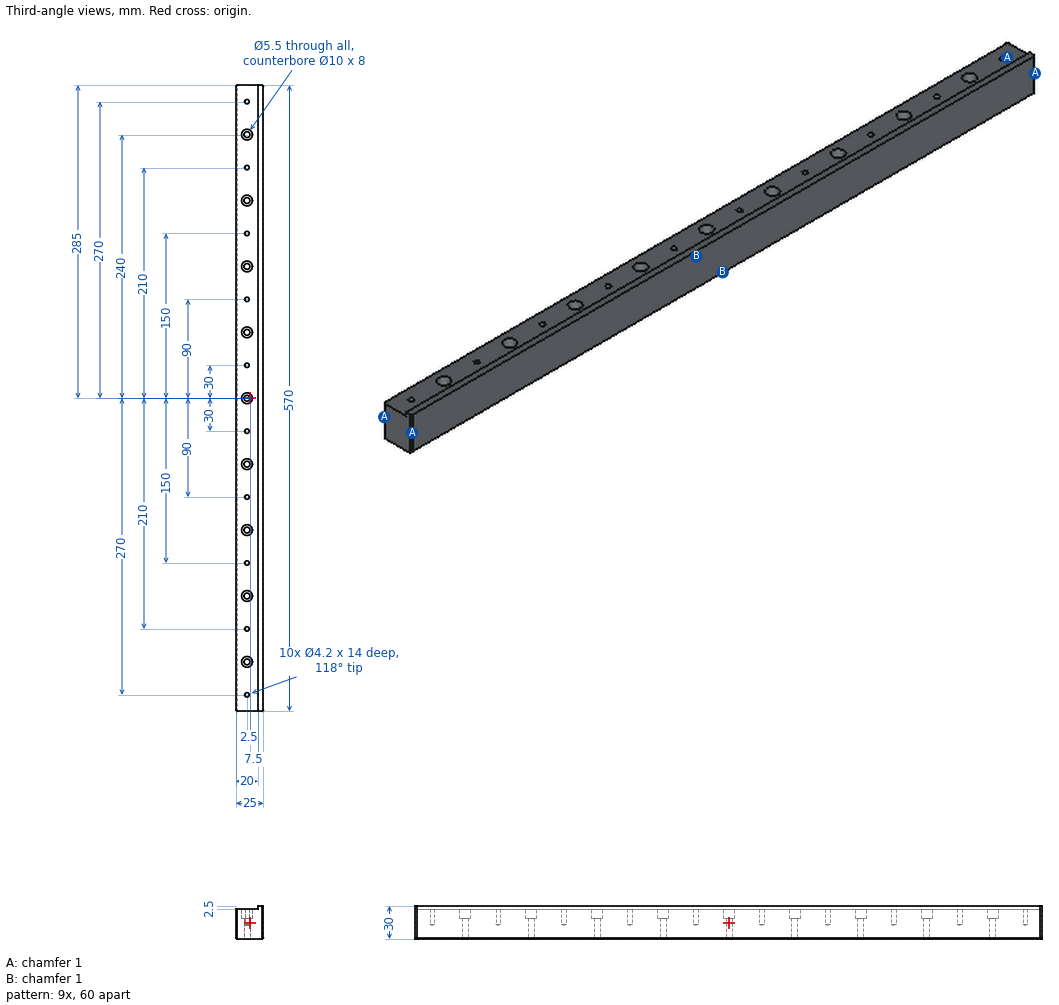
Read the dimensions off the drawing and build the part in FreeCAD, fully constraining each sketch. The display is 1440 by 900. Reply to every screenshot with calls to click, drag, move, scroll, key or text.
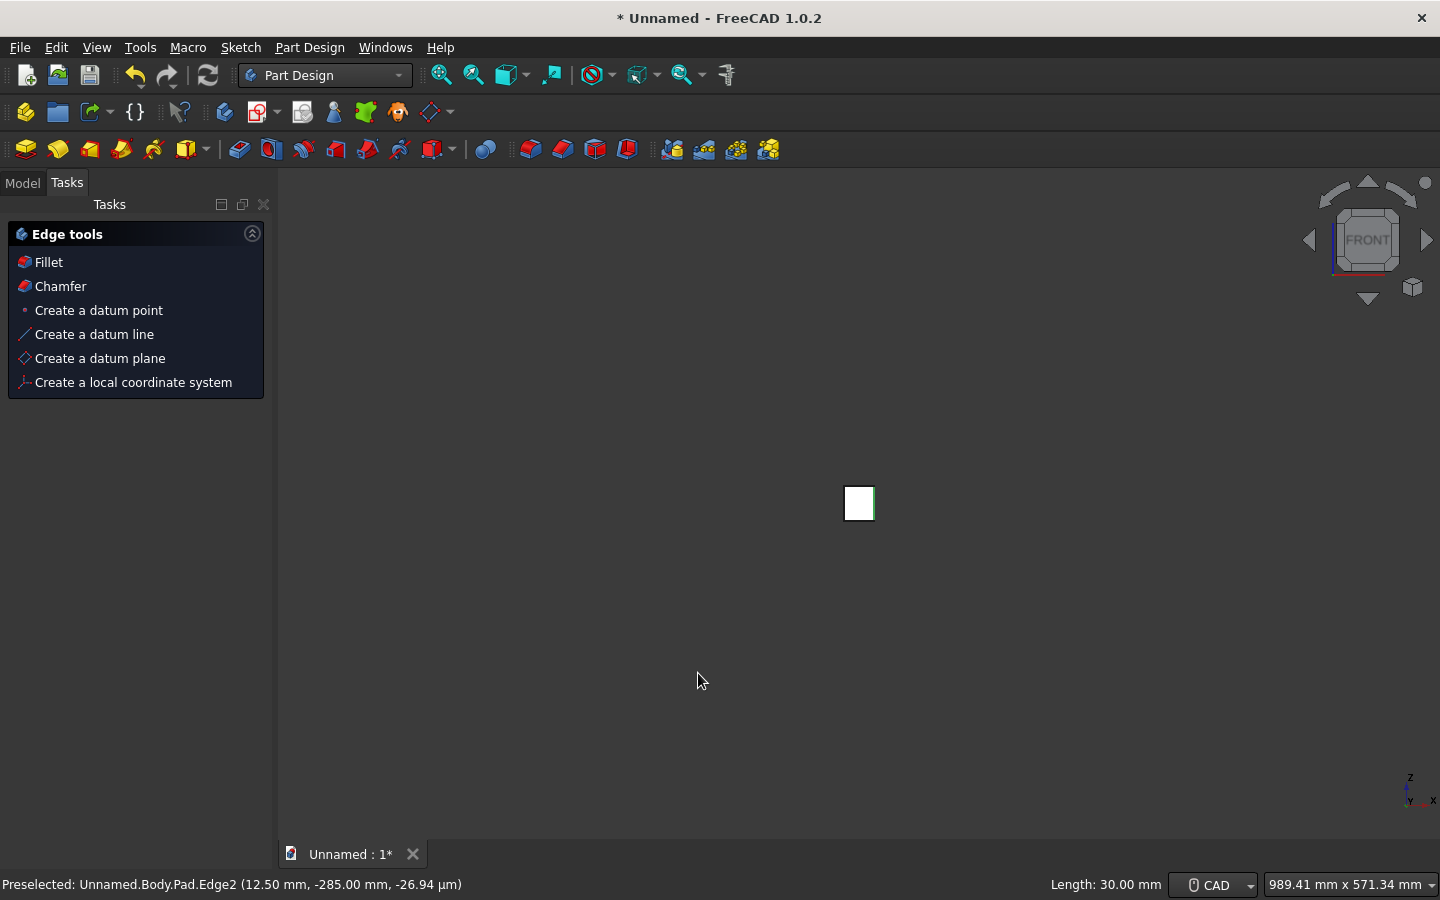
click(442, 76)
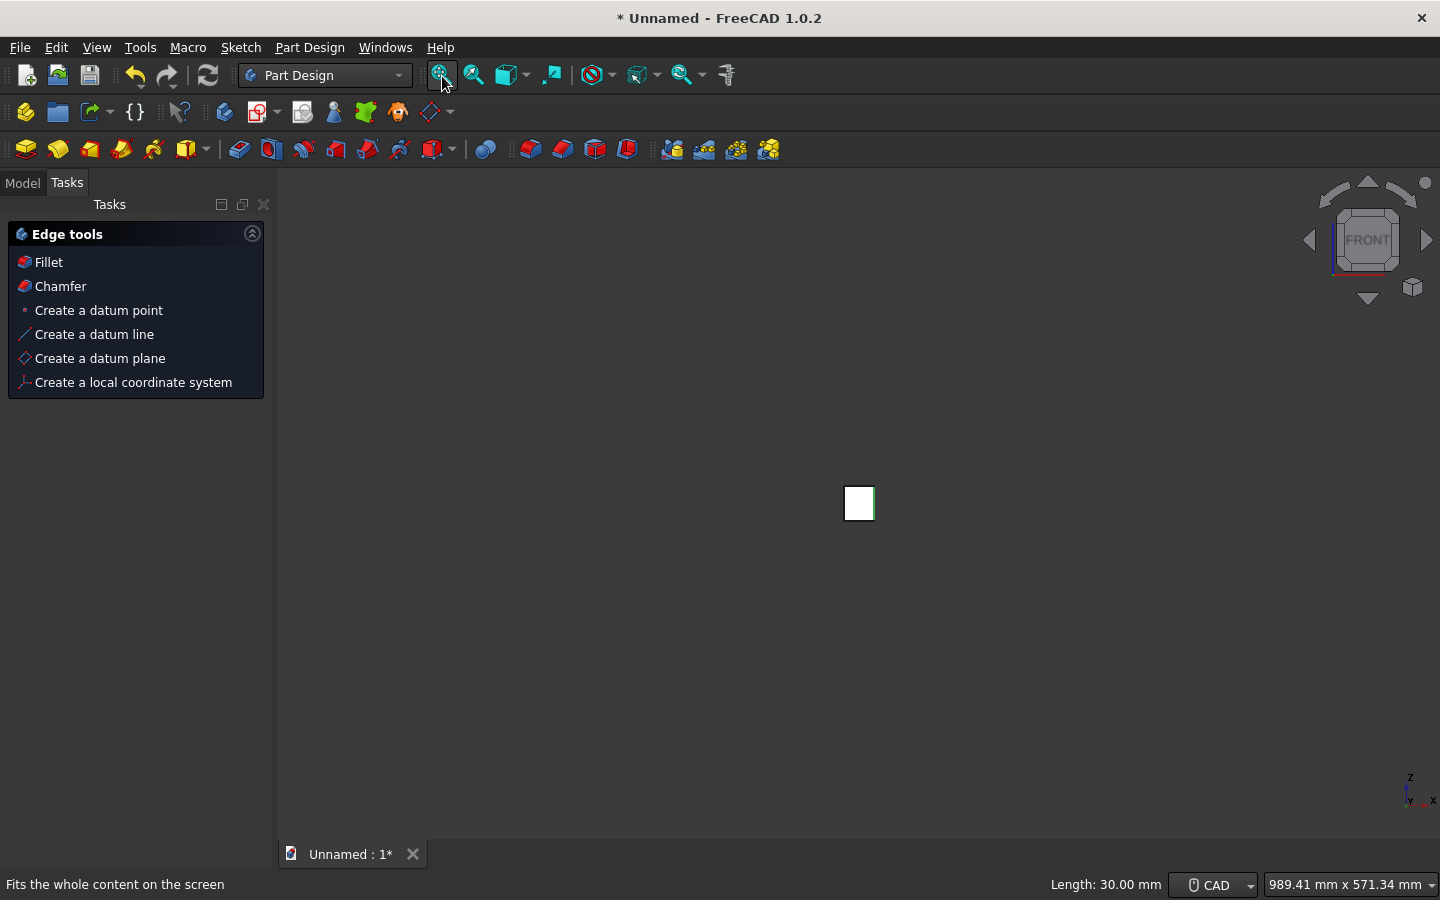
click(844, 503, ctrl)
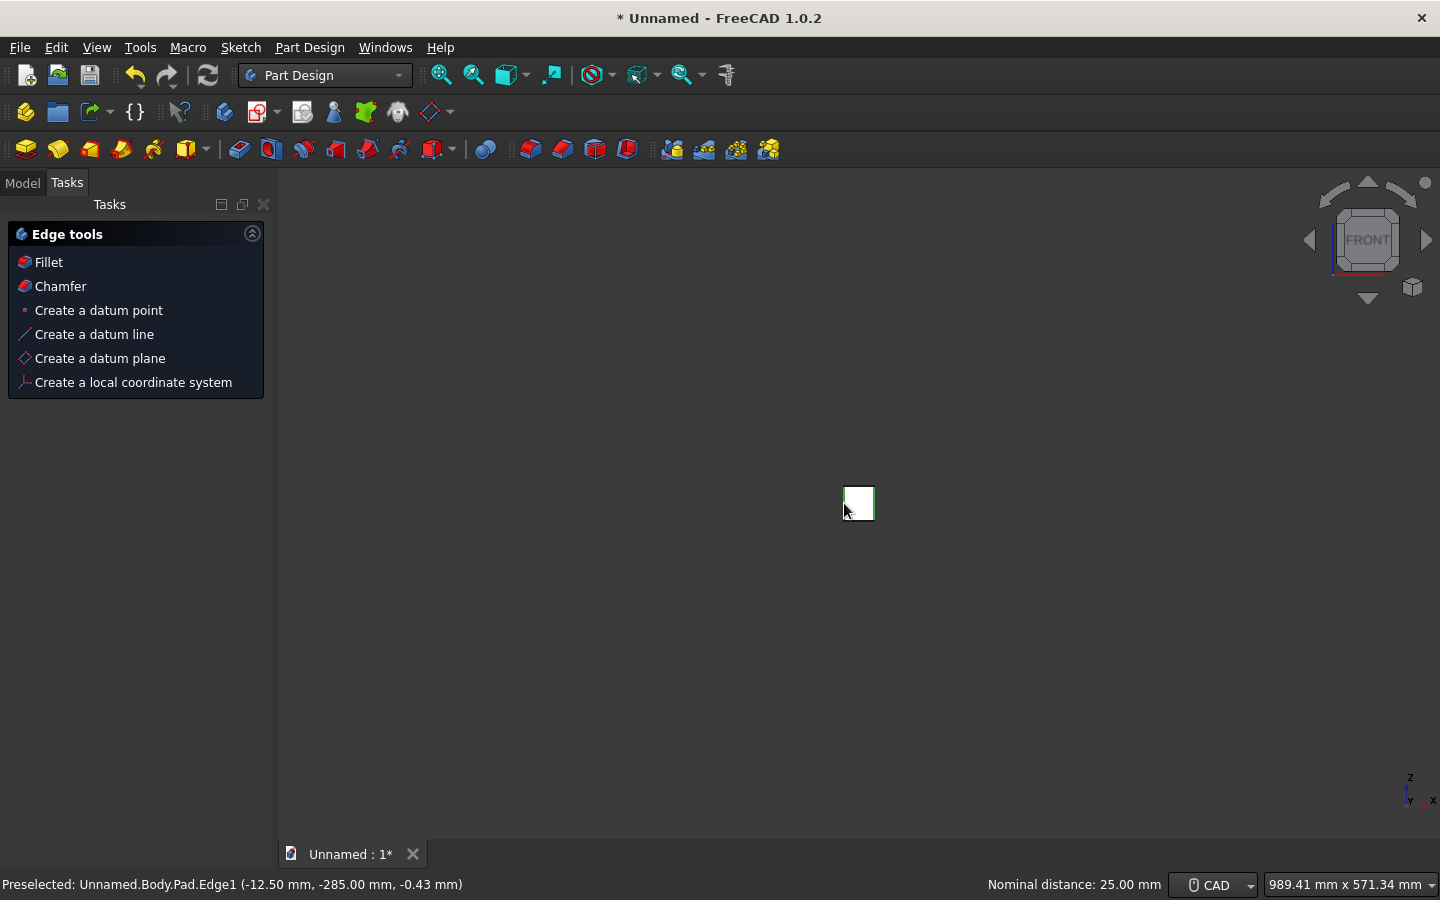
key(3)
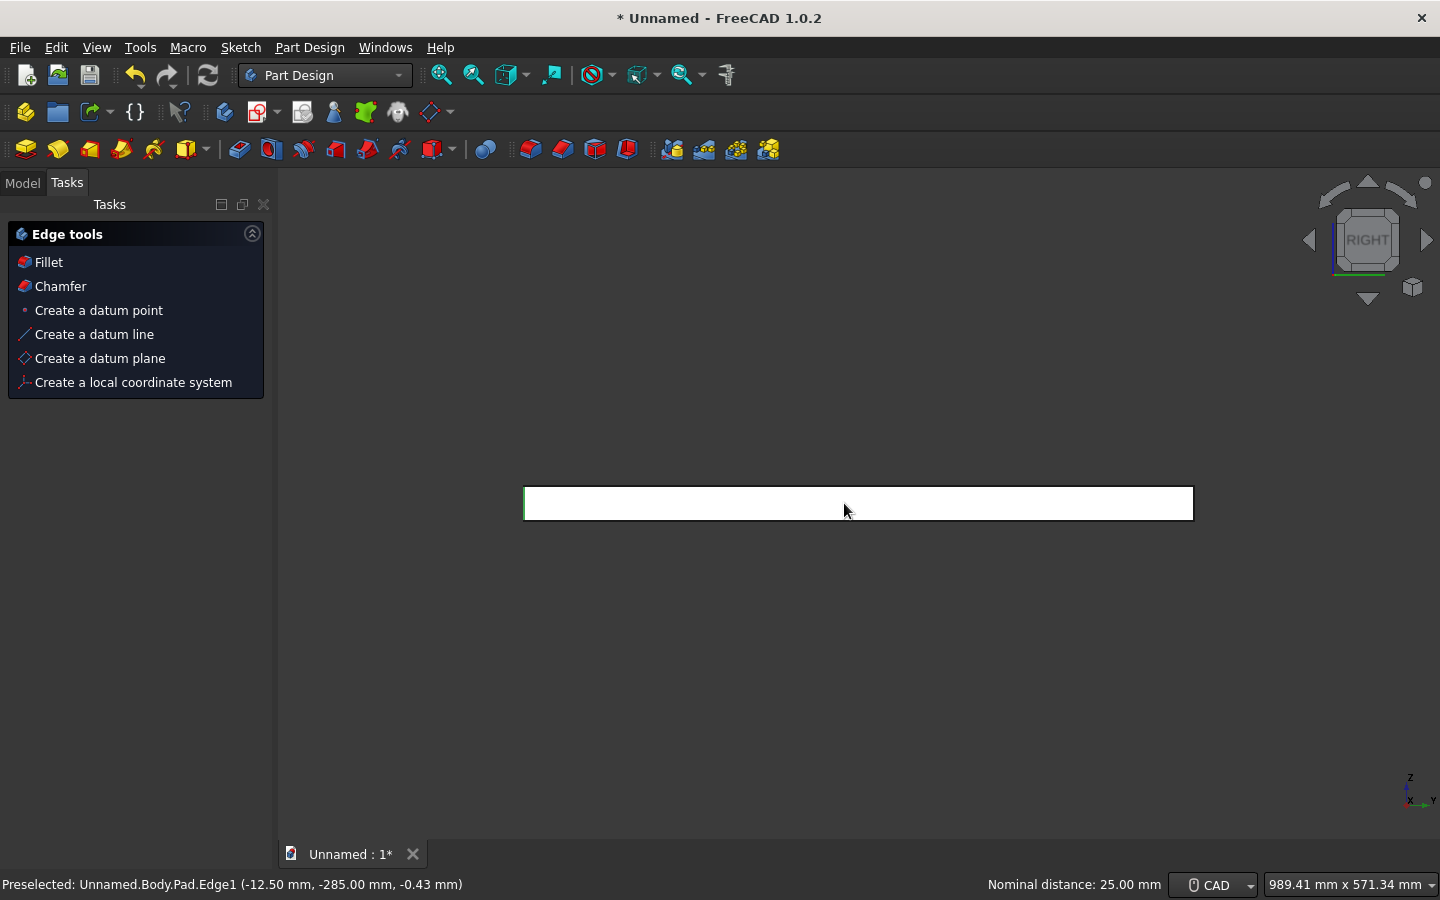
click(1194, 502, ctrl)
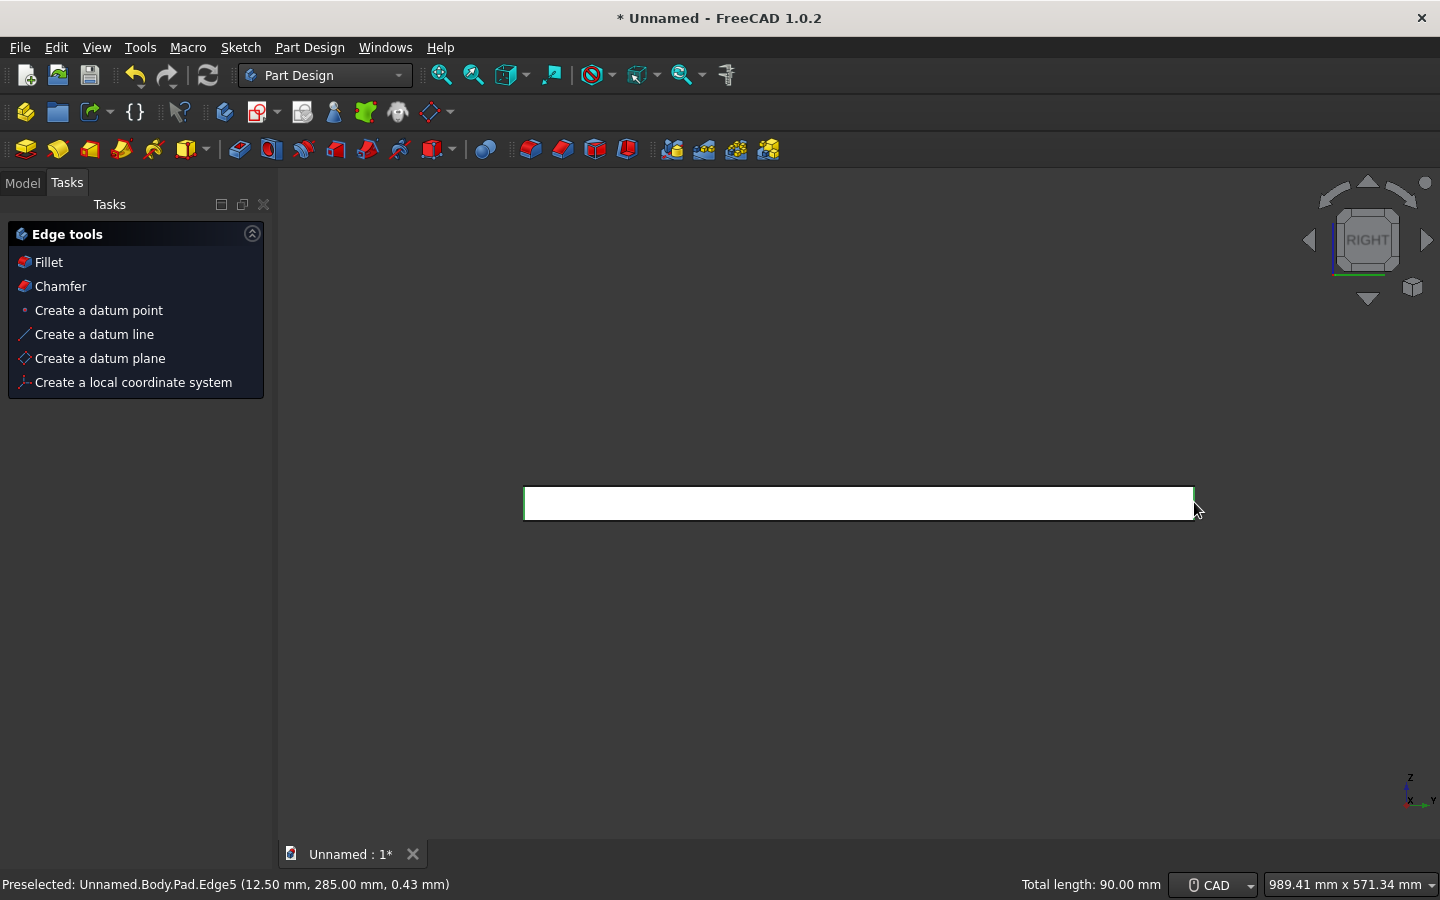
key(5)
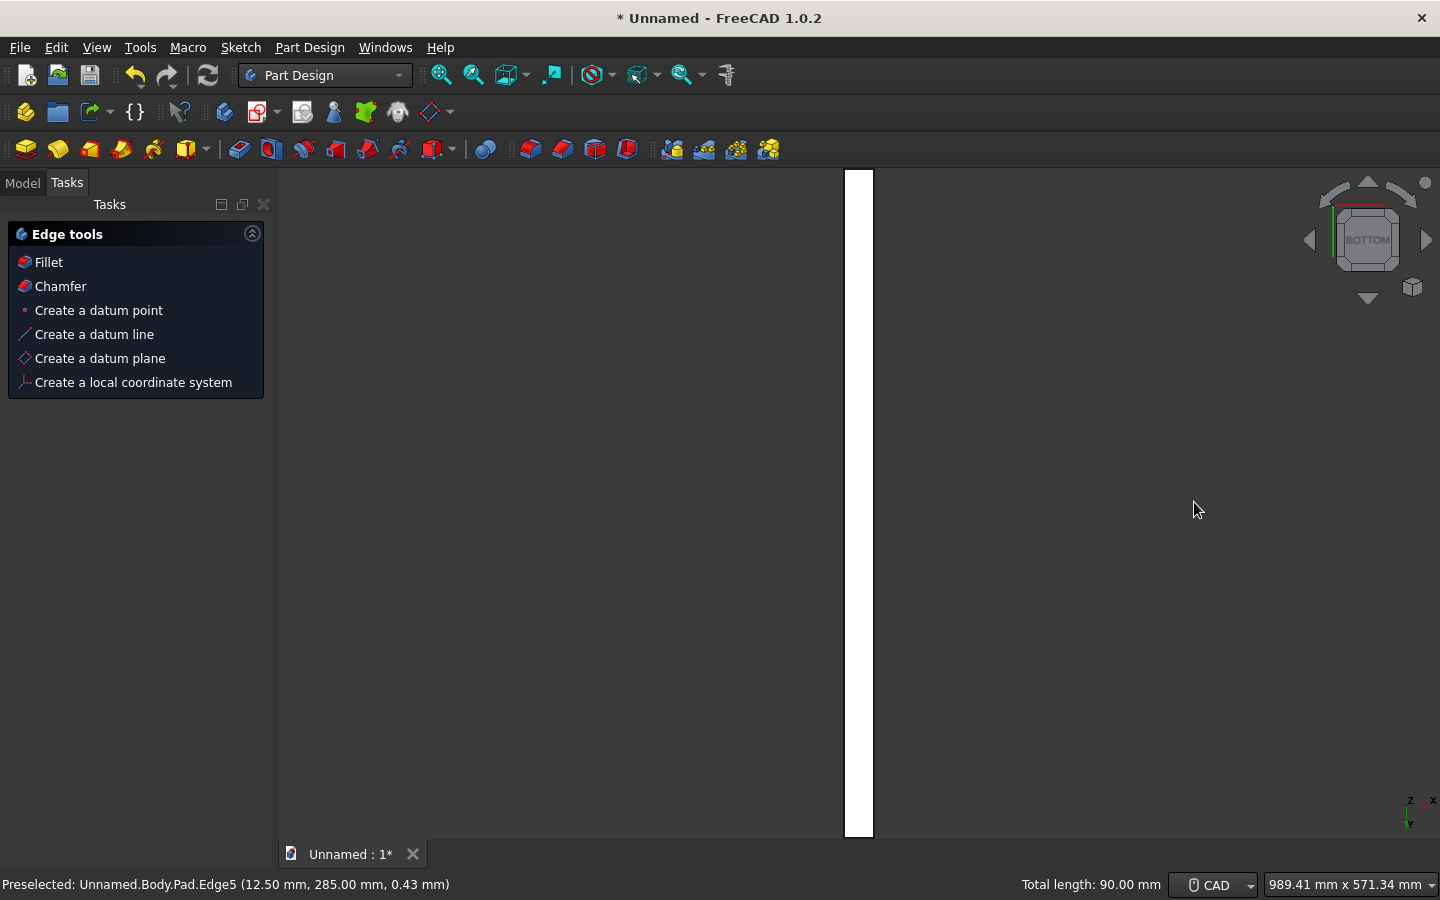
key(4)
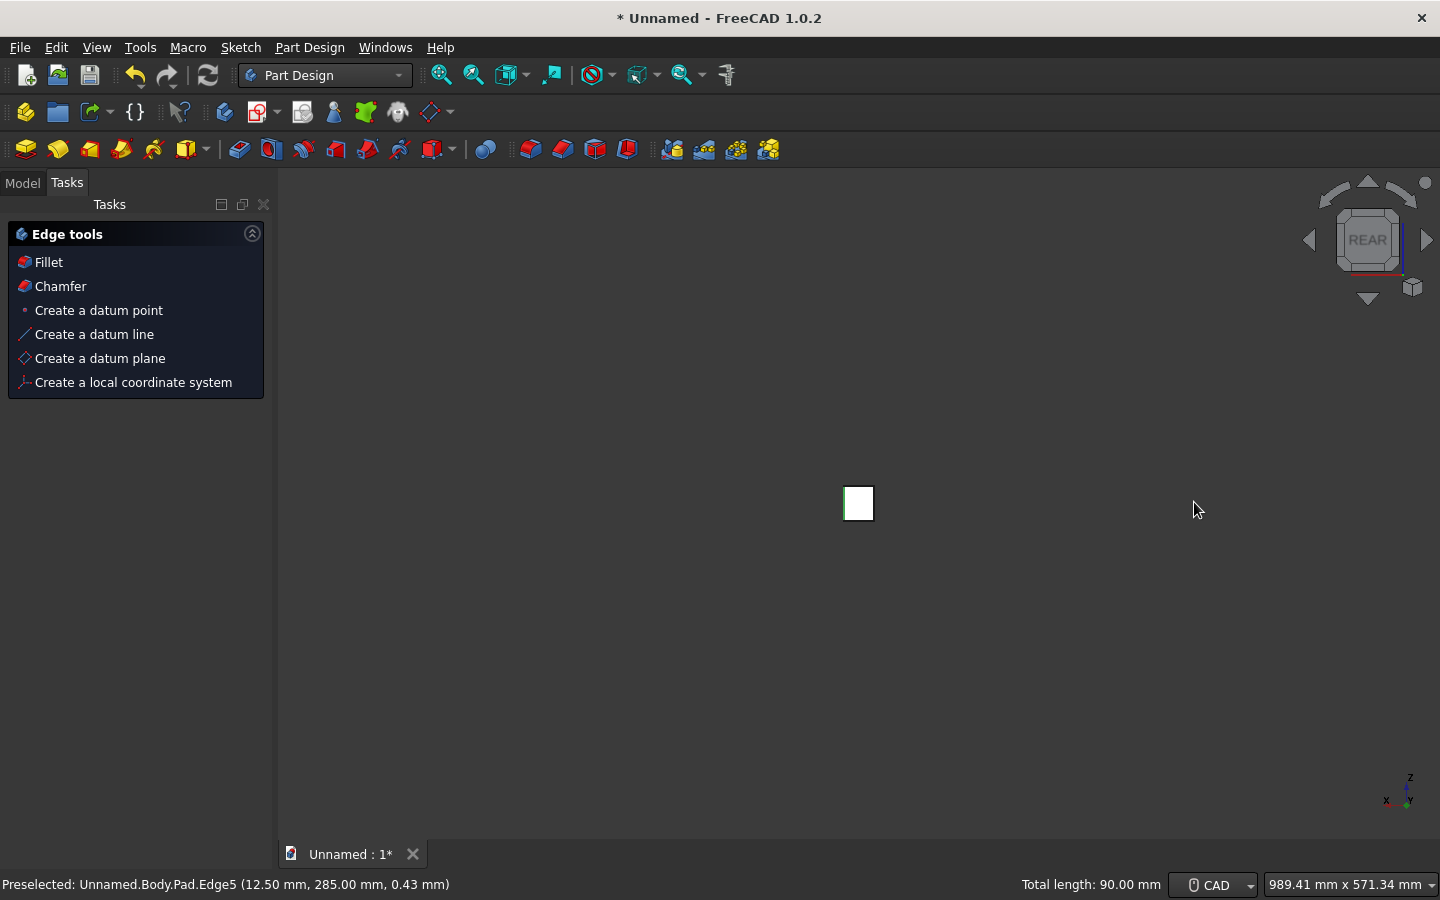
key(v)
key(f)